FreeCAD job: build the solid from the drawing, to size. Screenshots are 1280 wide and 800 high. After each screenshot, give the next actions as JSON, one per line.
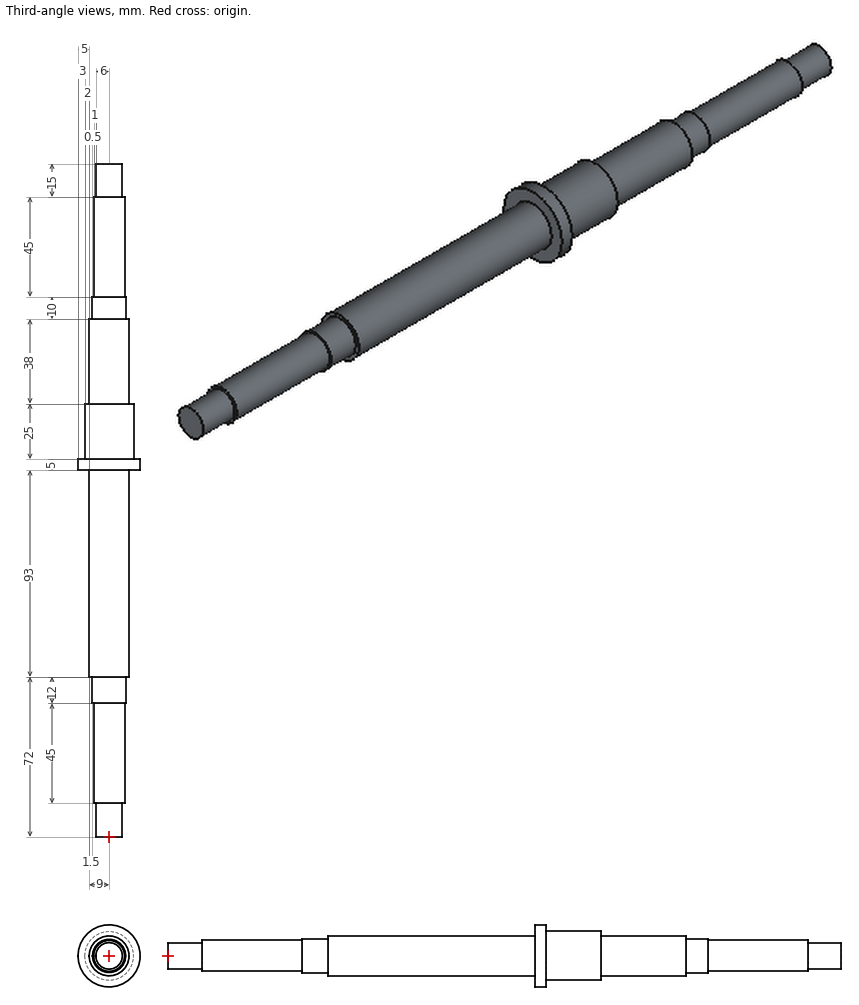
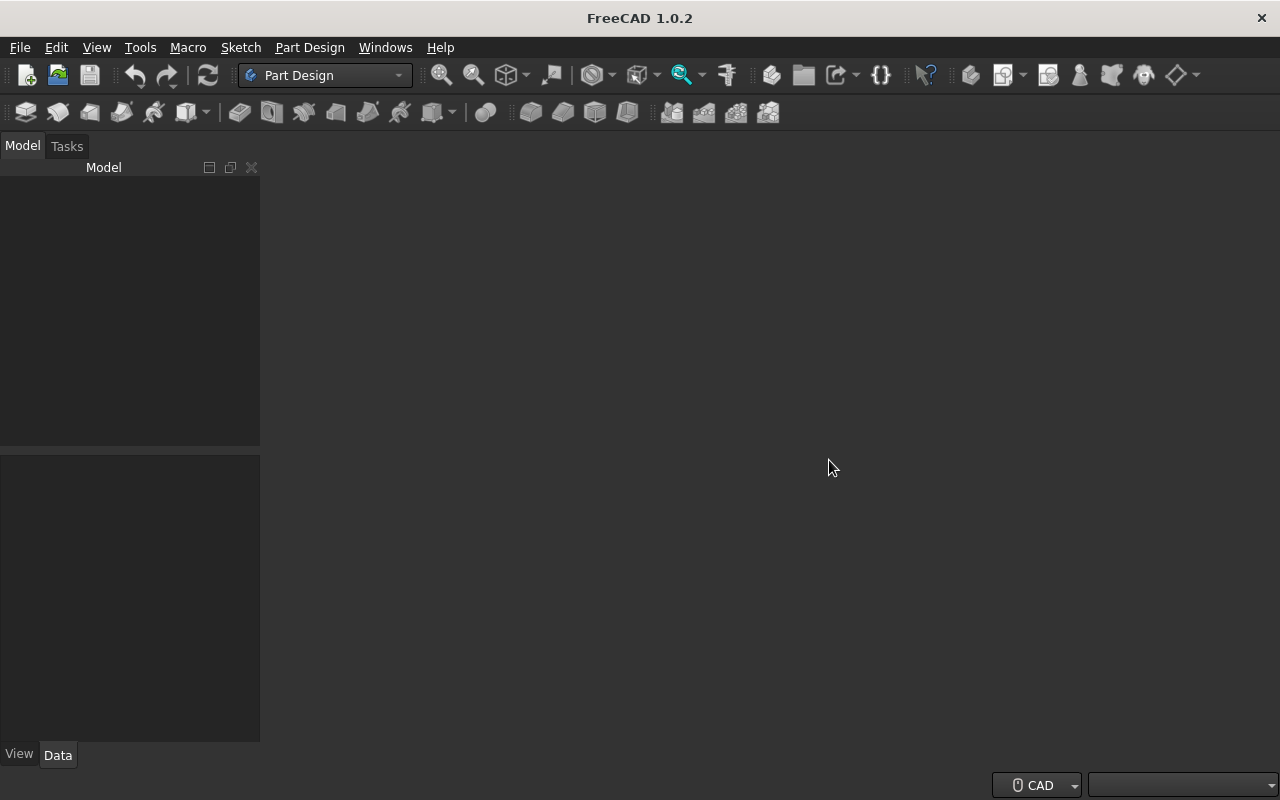
{"action": "key", "text": "ctrl+n"}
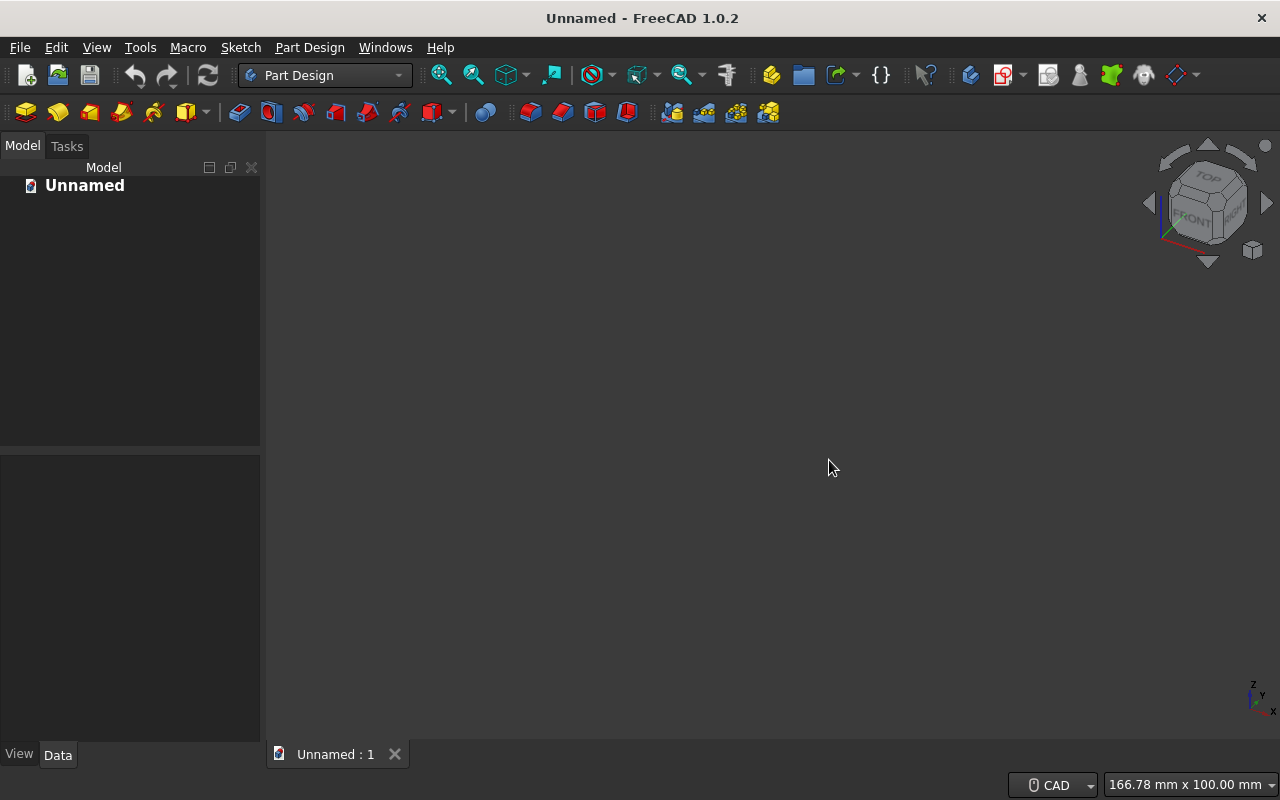
{"action": "left_click", "coordinate": [1004, 76]}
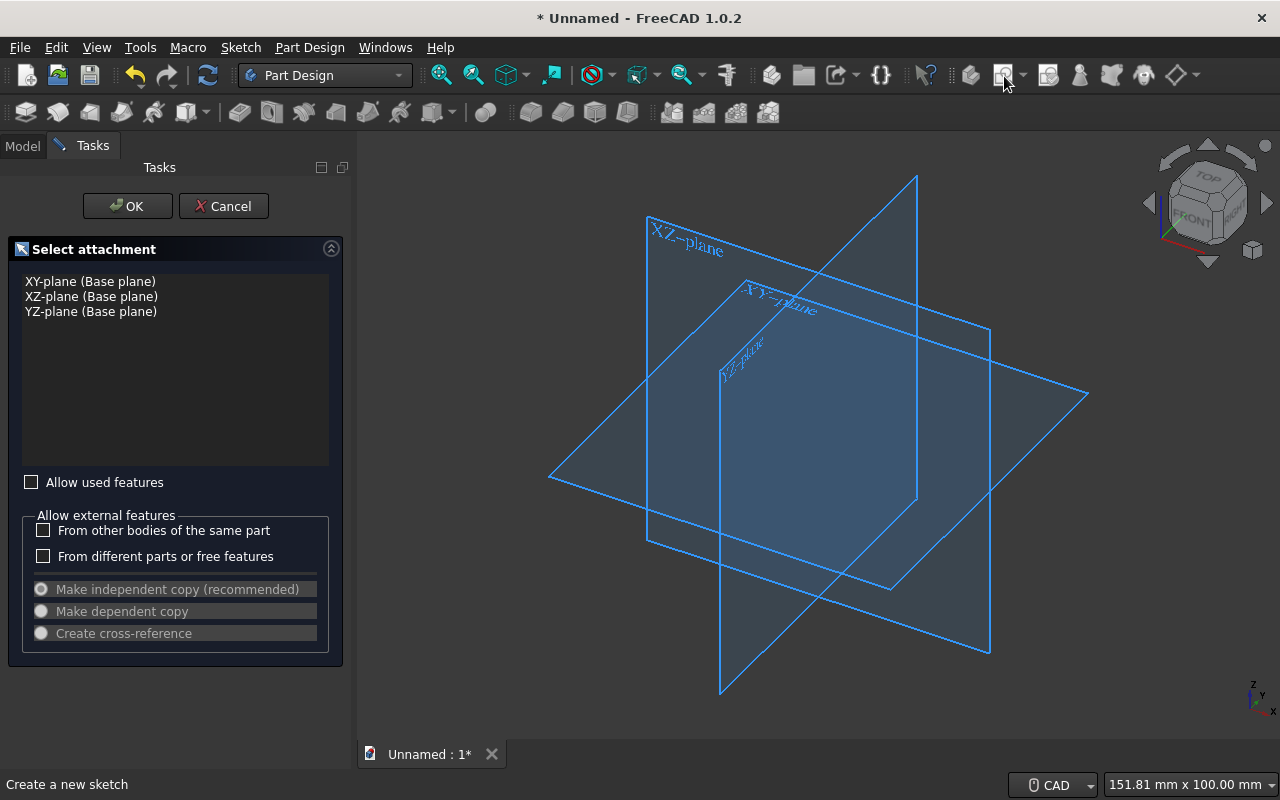
{"action": "left_click", "coordinate": [82, 282]}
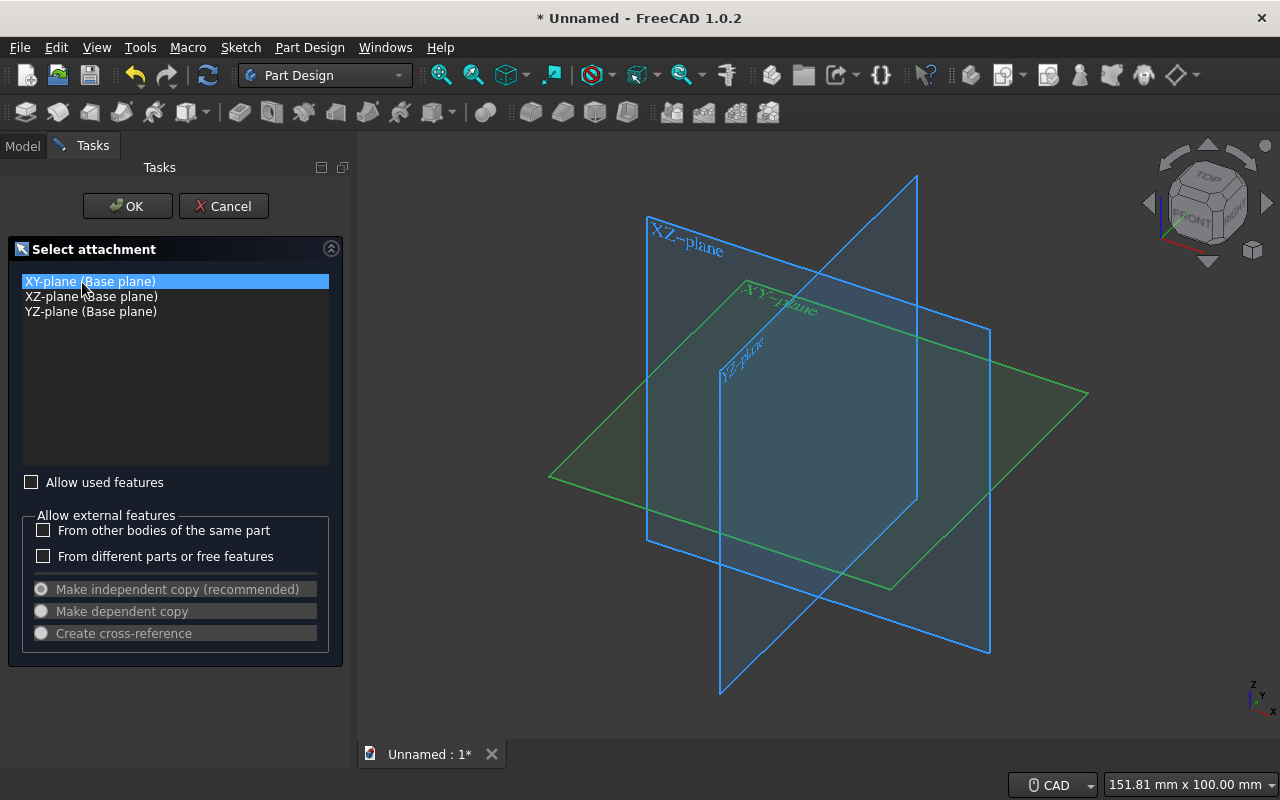
{"action": "left_click", "coordinate": [128, 206]}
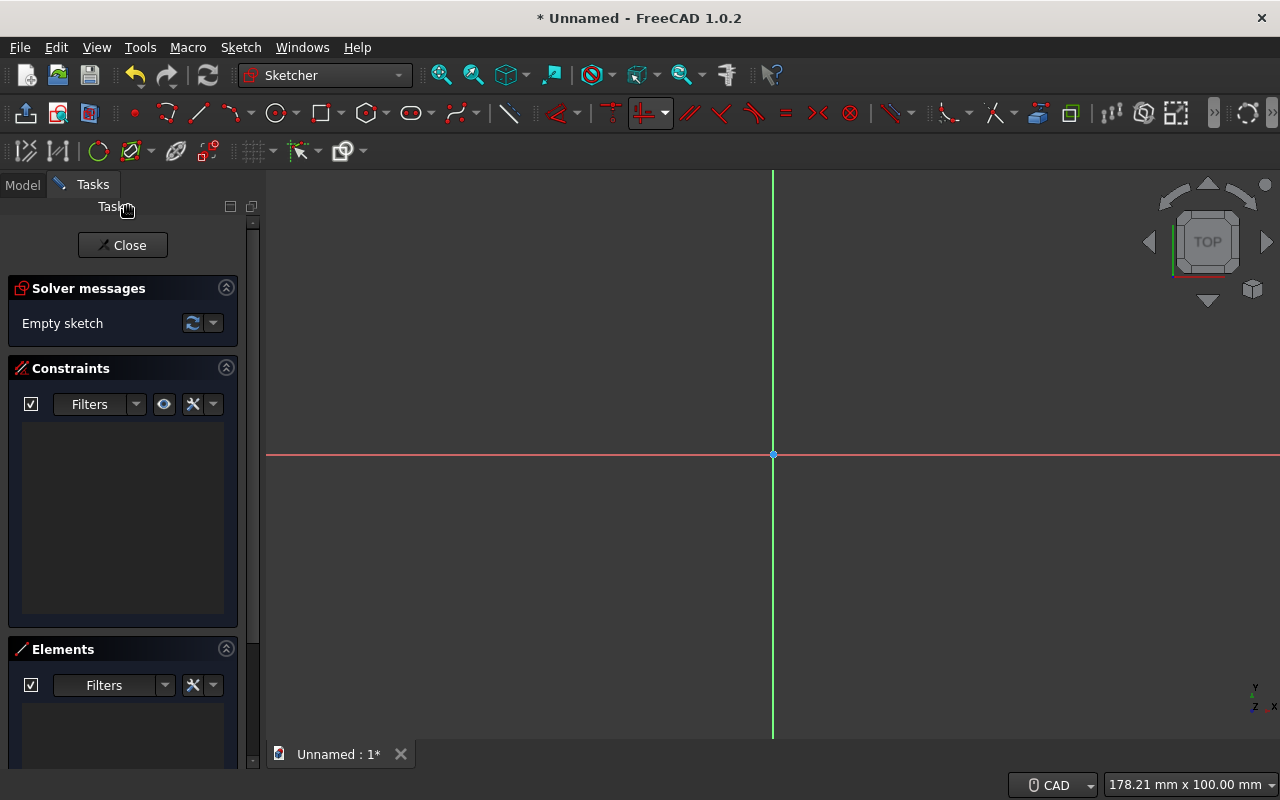
{"action": "scroll", "coordinate": [697, 673], "scroll_direction": "down", "scroll_amount": 8}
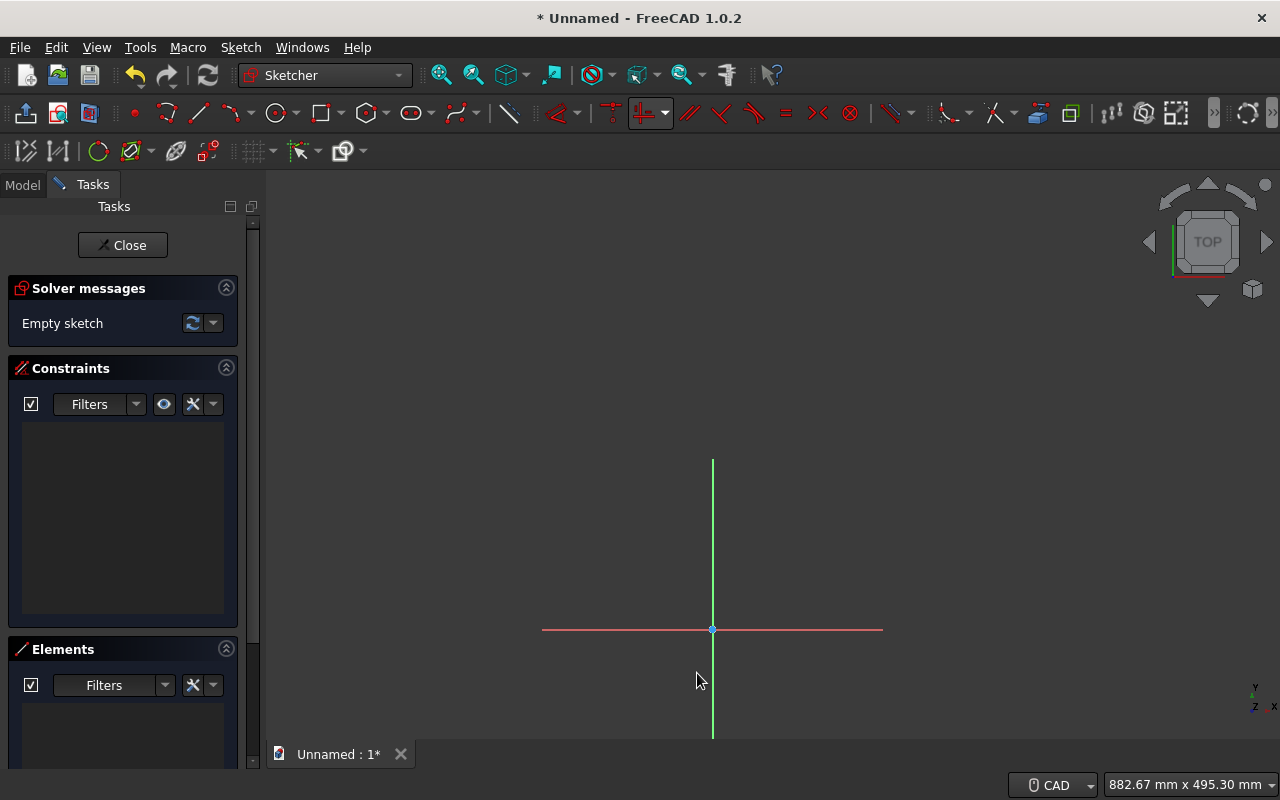
{"action": "key", "text": "g m"}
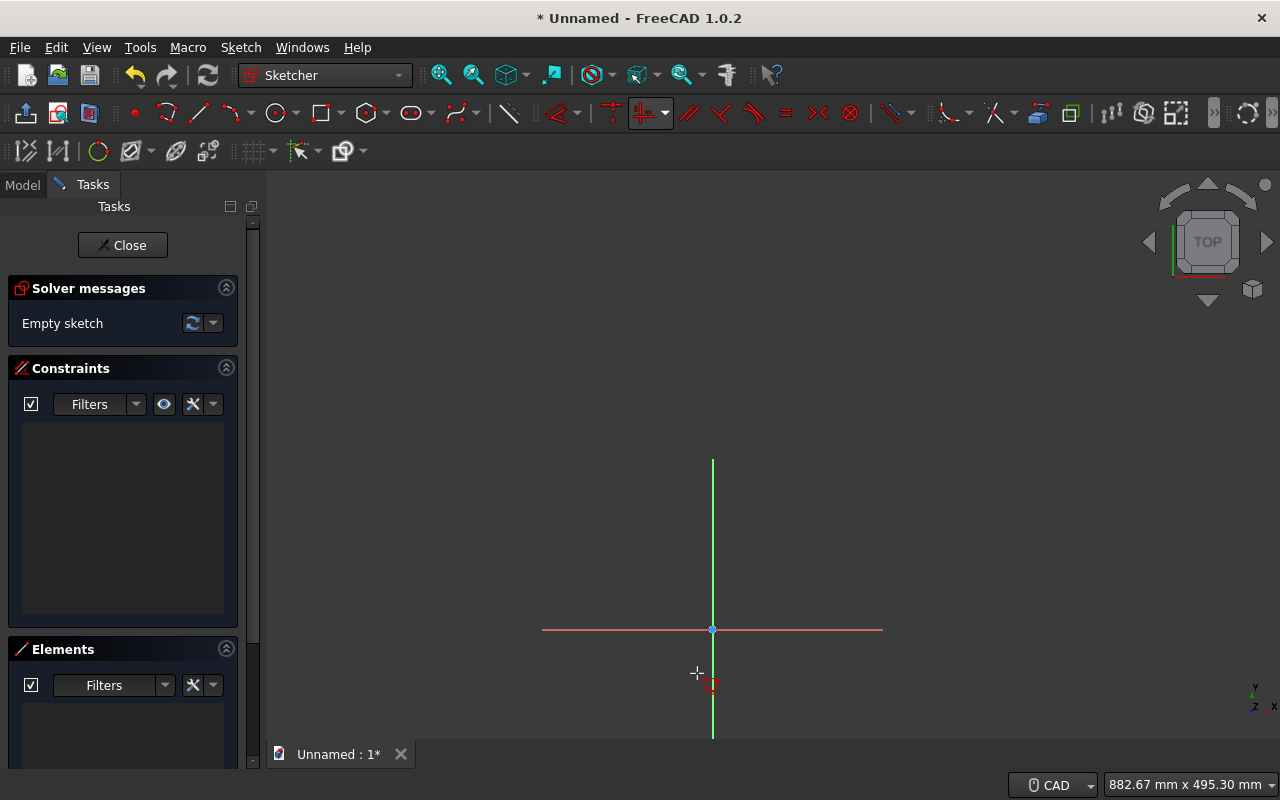
{"action": "left_click", "coordinate": [713, 630]}
{"action": "left_click", "coordinate": [704, 282]}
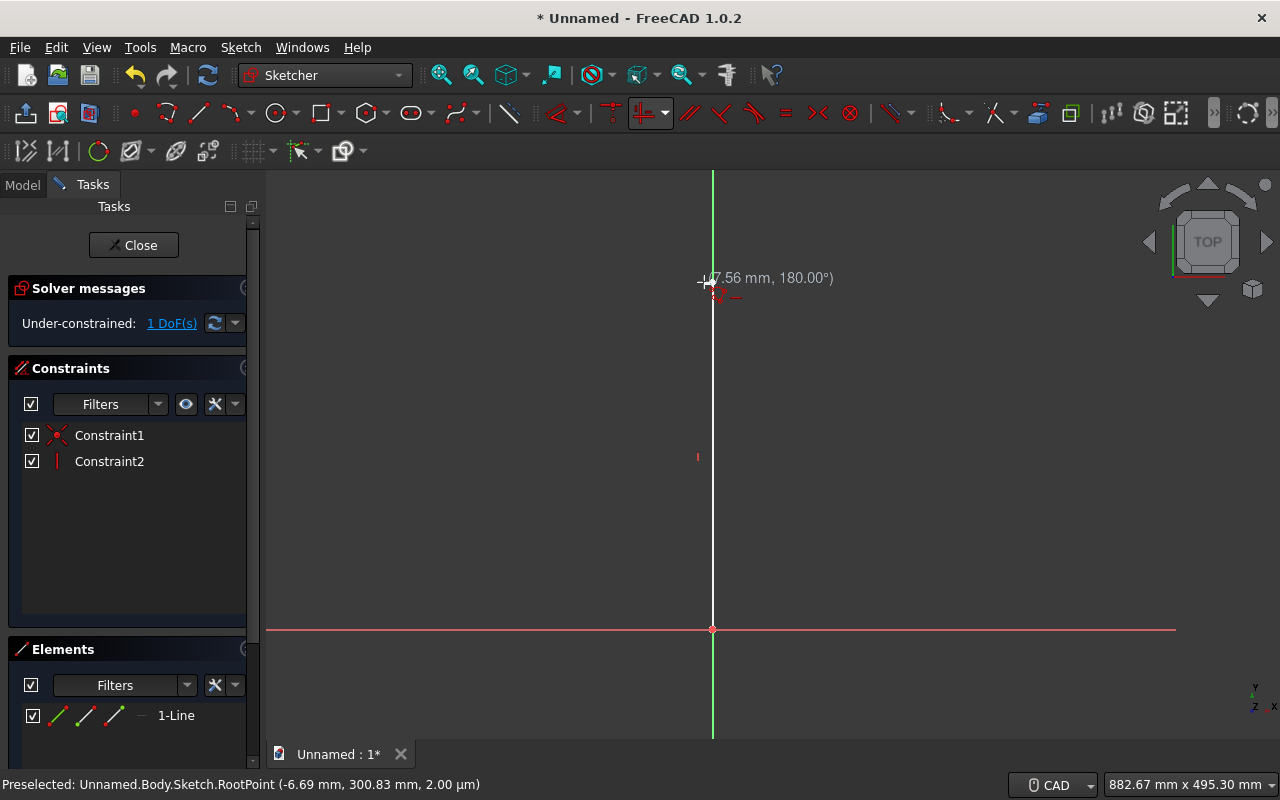
{"action": "scroll", "coordinate": [706, 282], "scroll_direction": "up", "scroll_amount": 5}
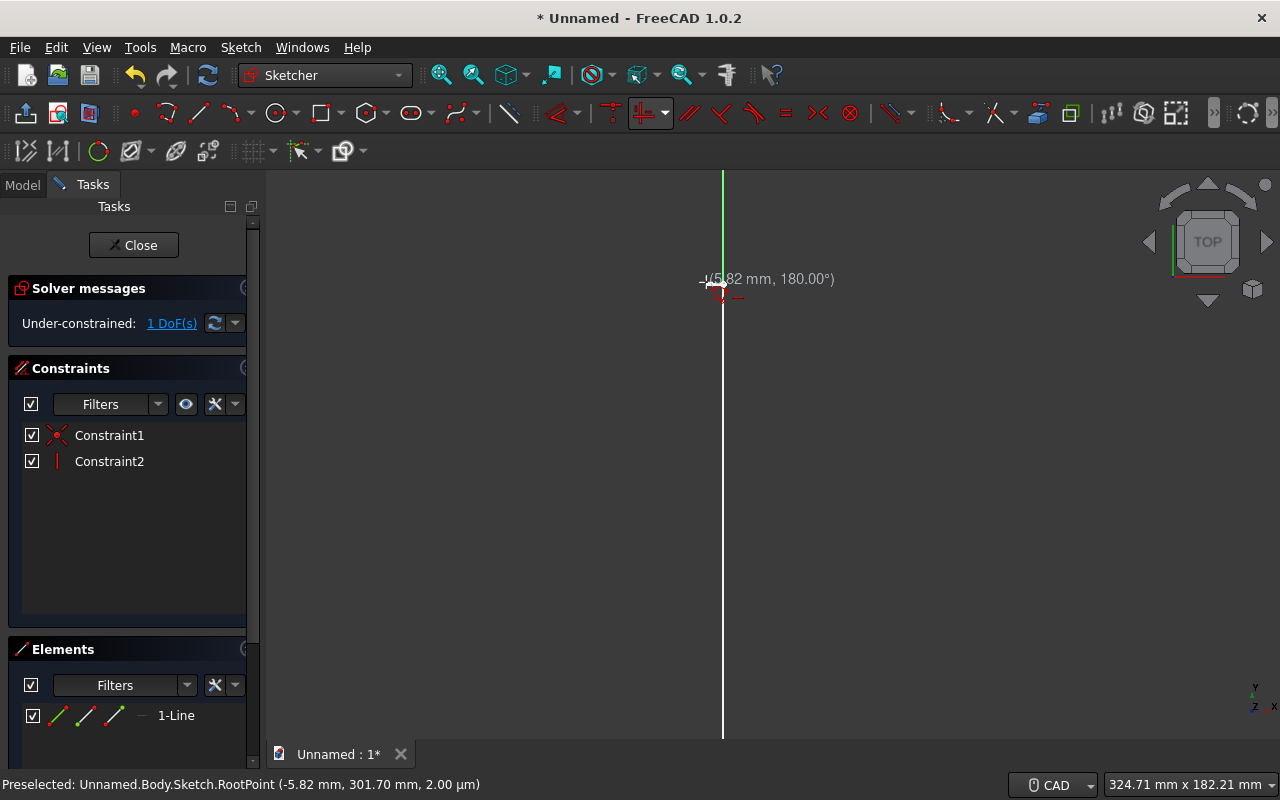
{"action": "left_click", "coordinate": [705, 282]}
{"action": "left_click", "coordinate": [705, 327]}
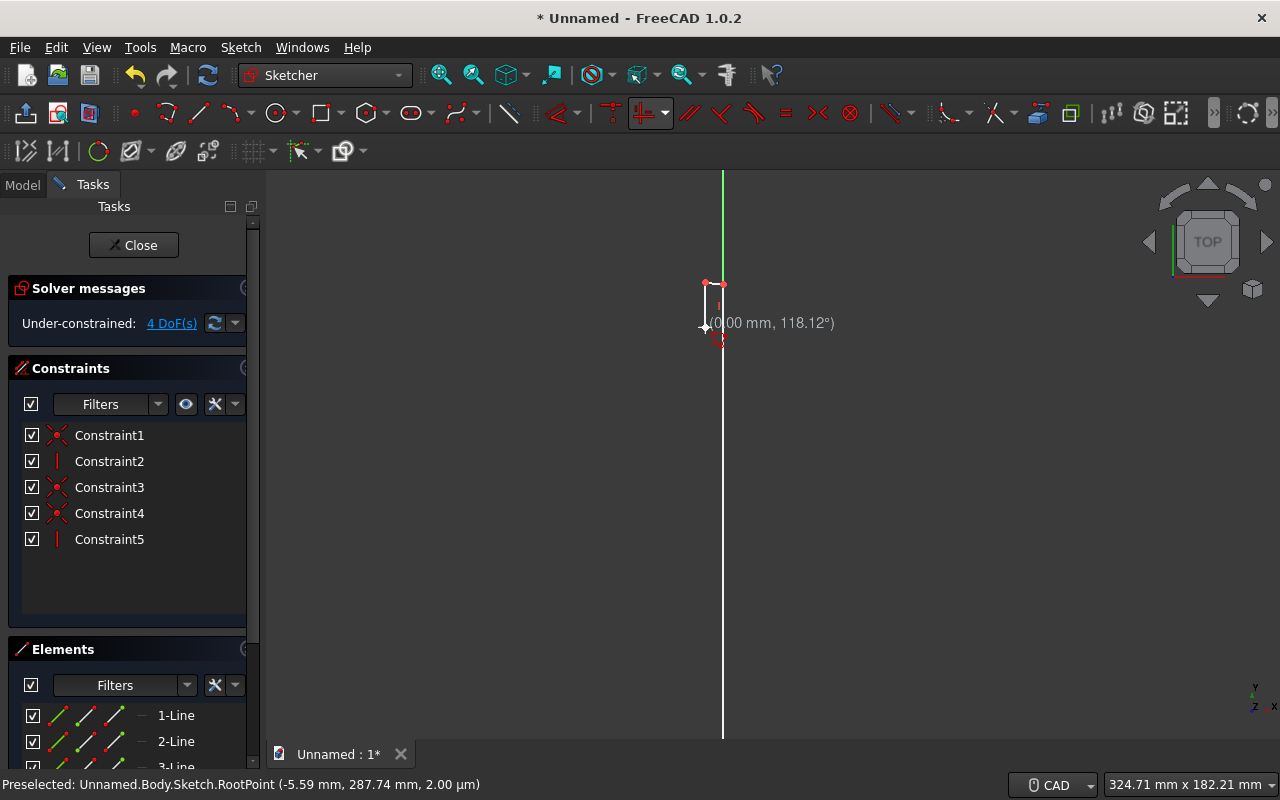
{"action": "scroll", "coordinate": [702, 327], "scroll_direction": "up", "scroll_amount": 9}